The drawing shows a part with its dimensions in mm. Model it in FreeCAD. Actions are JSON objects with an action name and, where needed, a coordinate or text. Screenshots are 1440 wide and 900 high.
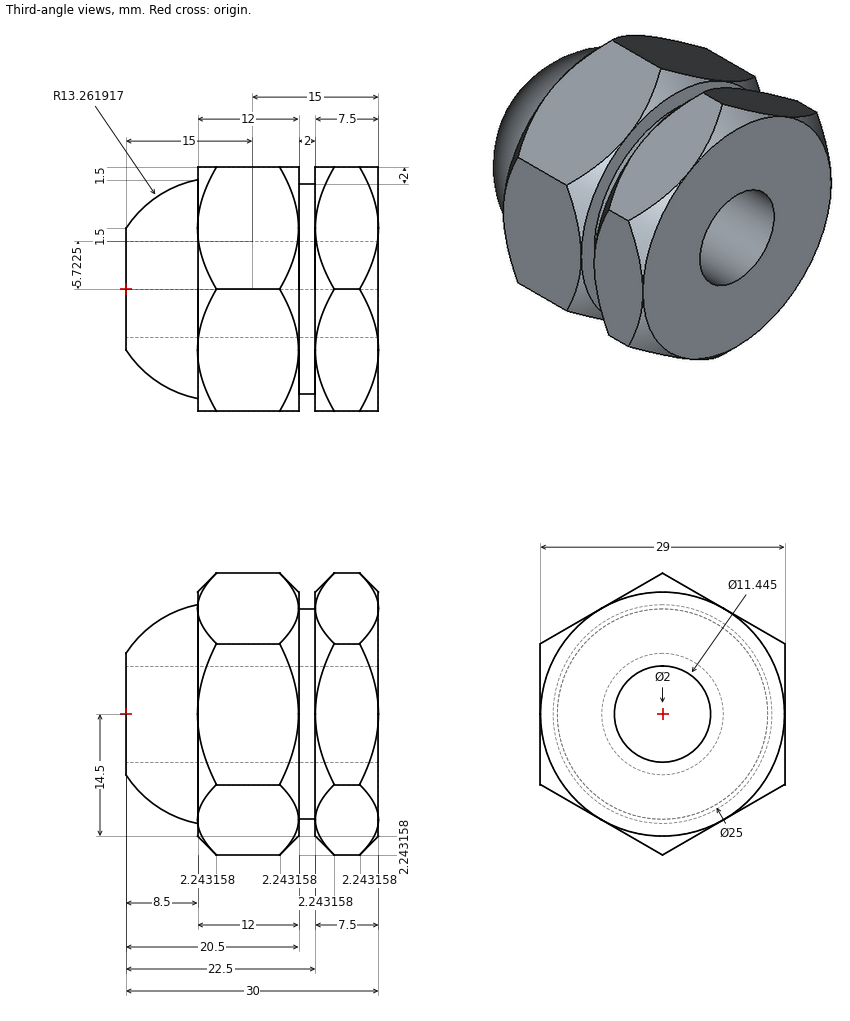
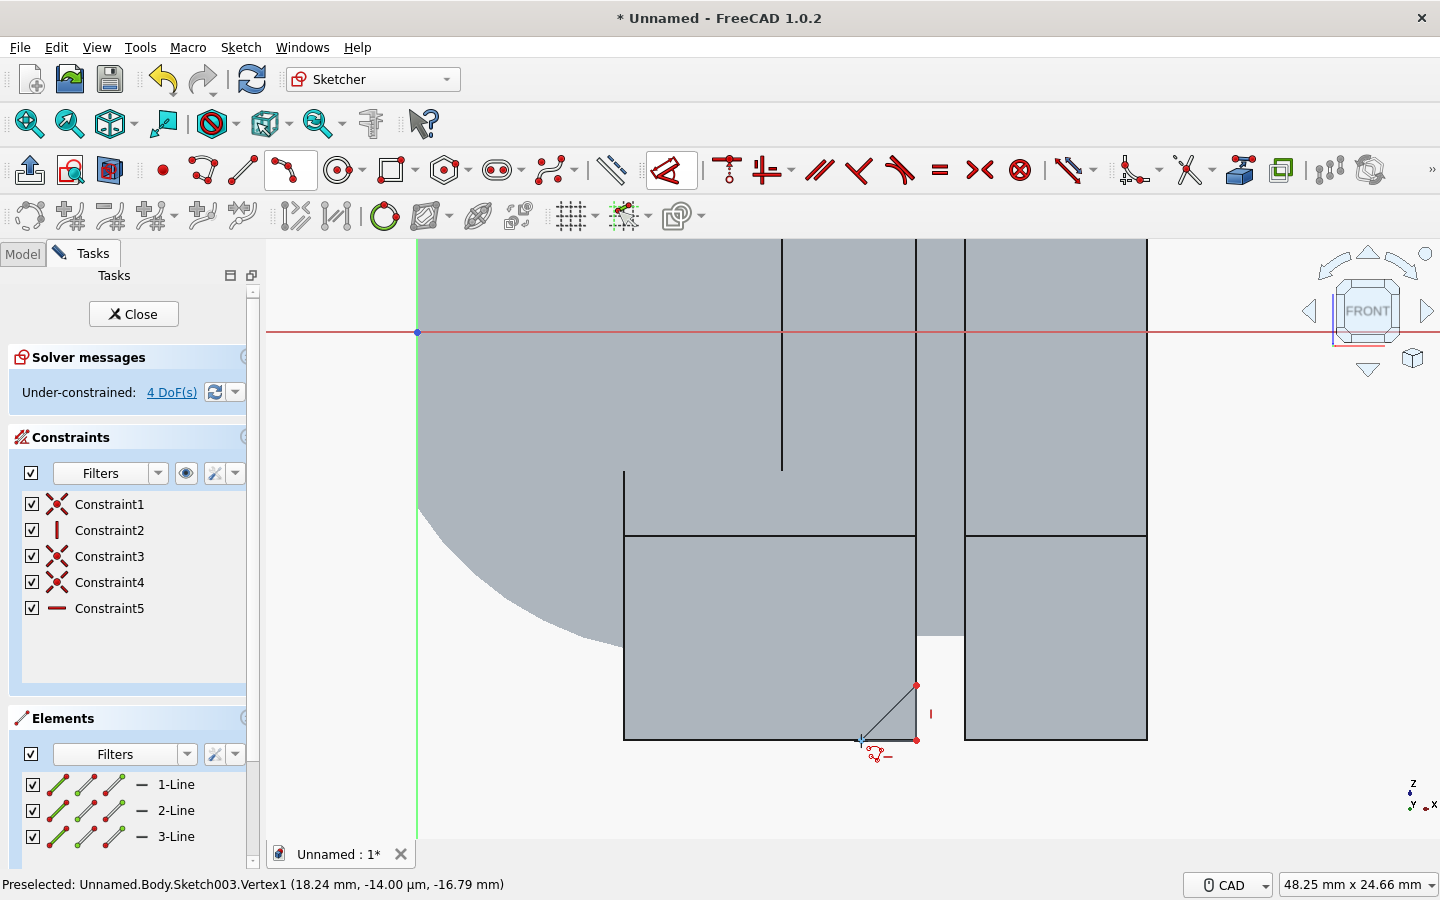
{"action": "left_click", "coordinate": [965, 685]}
{"action": "left_click", "coordinate": [1019, 740]}
{"action": "left_click", "coordinate": [965, 740]}
{"action": "left_click", "coordinate": [965, 686]}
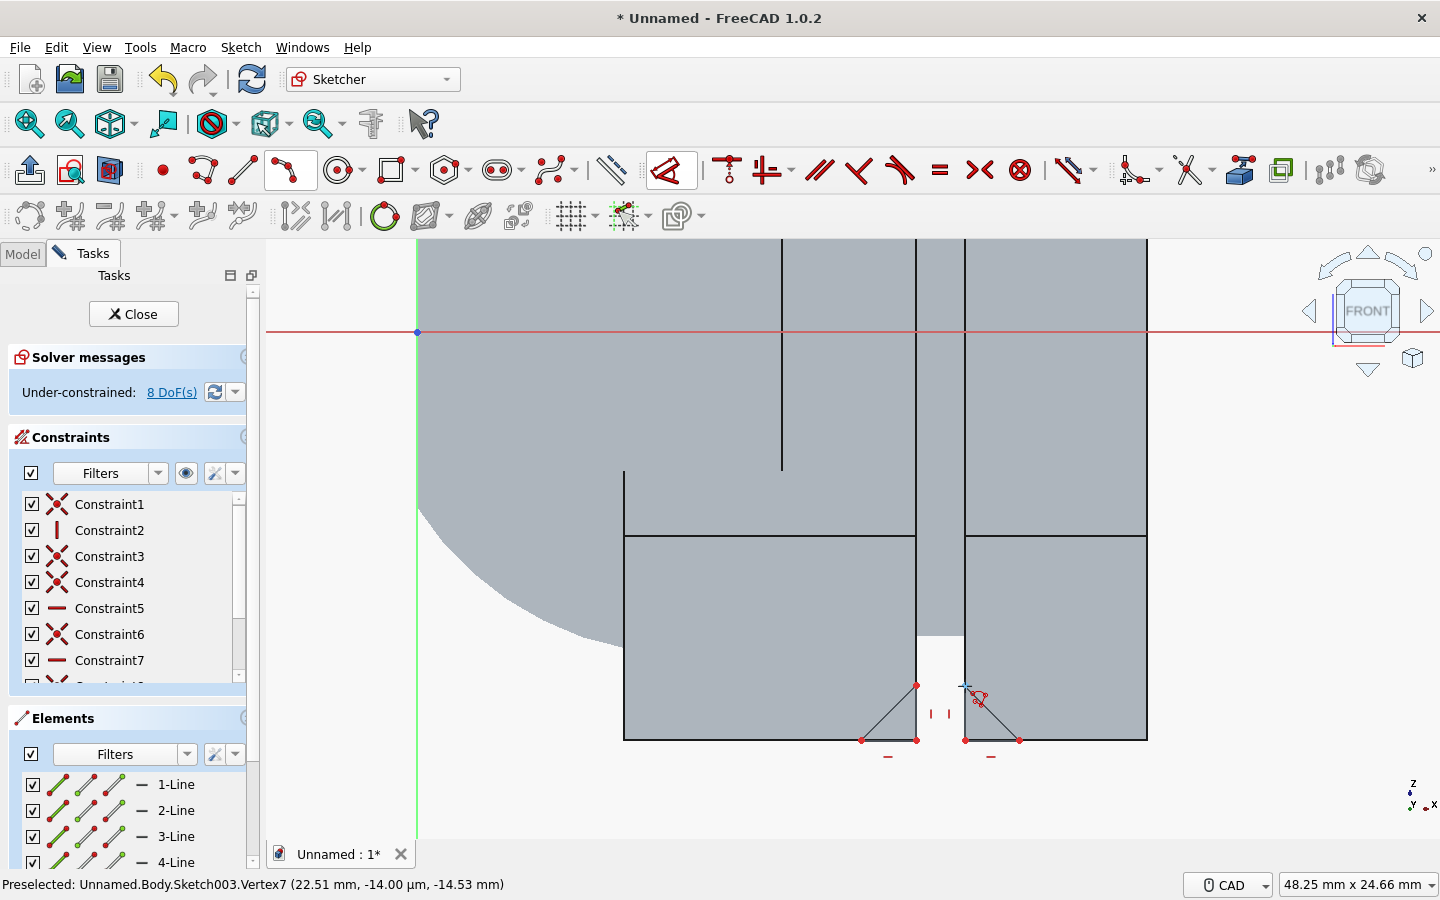
{"action": "left_click", "coordinate": [624, 685]}
{"action": "left_click", "coordinate": [679, 740]}
{"action": "left_click", "coordinate": [624, 740]}
{"action": "left_click", "coordinate": [624, 686]}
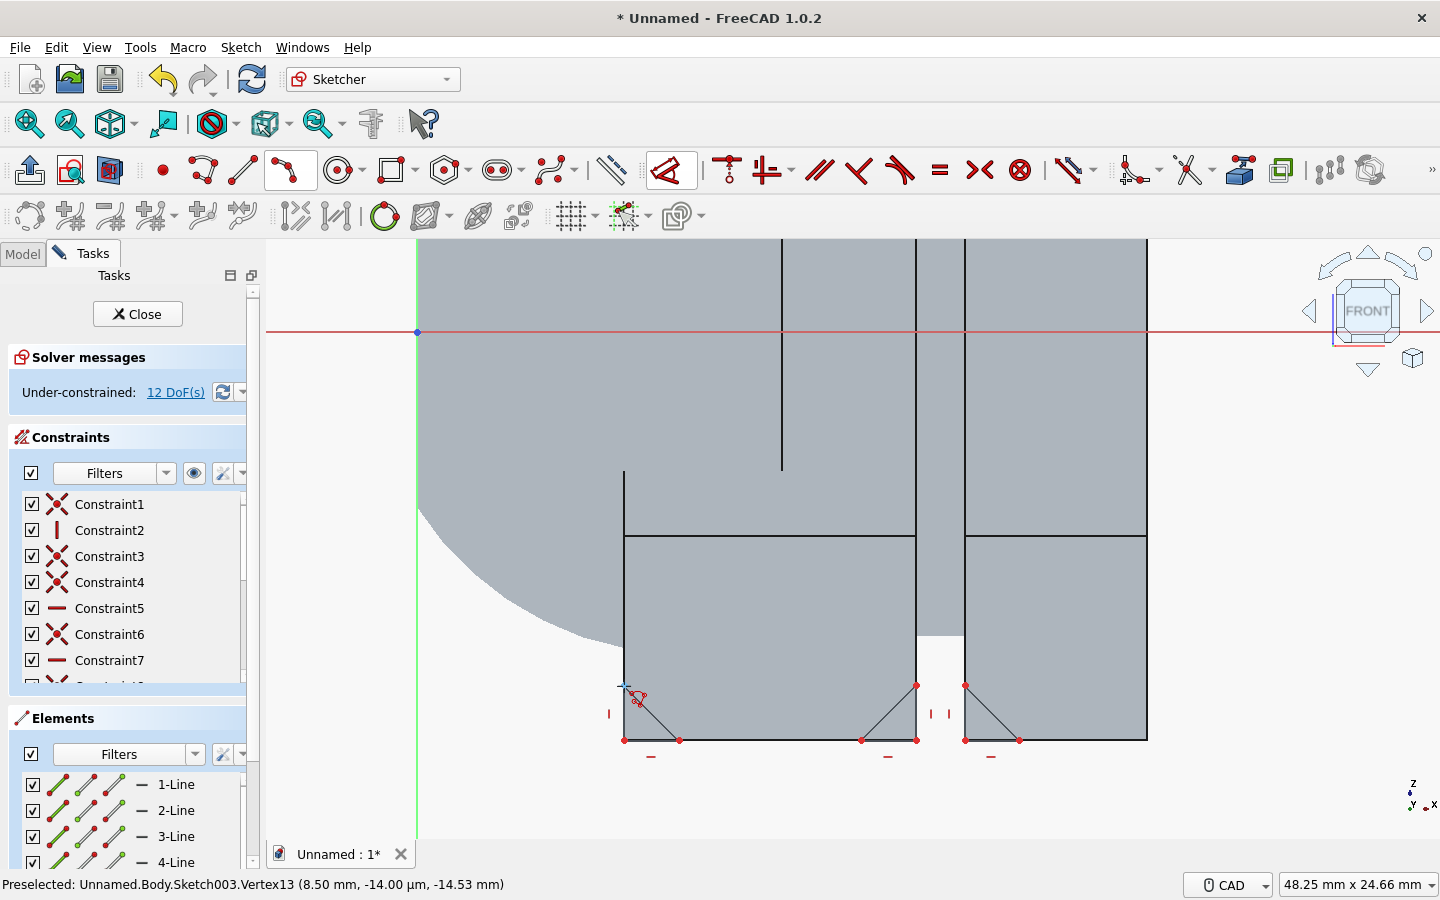
{"action": "left_click", "coordinate": [1093, 740]}
{"action": "left_click", "coordinate": [1147, 685]}
{"action": "left_click", "coordinate": [1147, 740]}
{"action": "left_click", "coordinate": [1093, 741]}
{"action": "key", "text": "Escape"}
{"action": "key", "text": "Escape"}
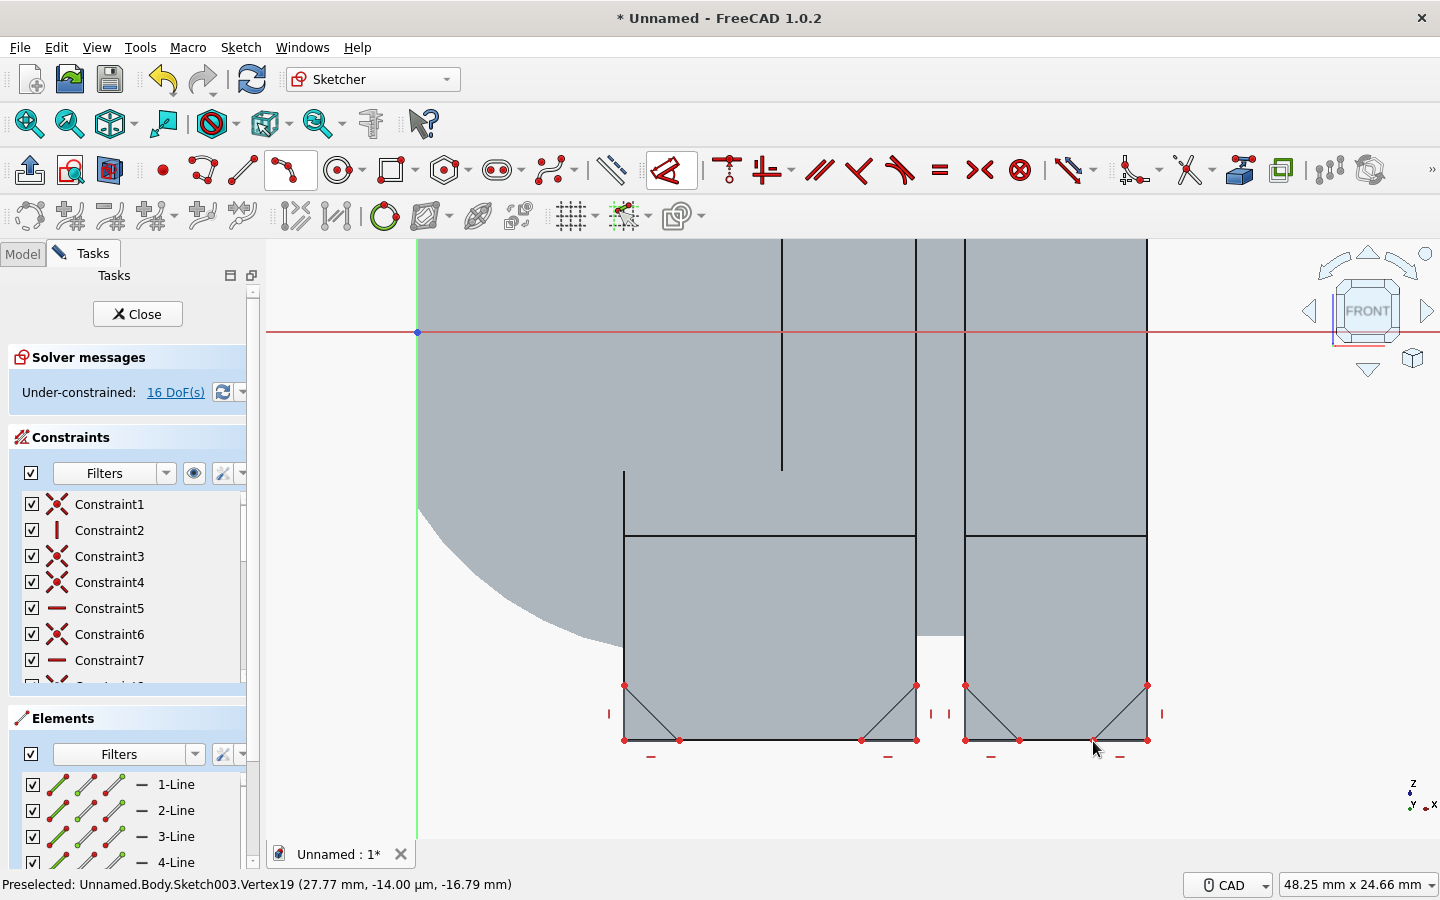
{"action": "left_click", "coordinate": [1147, 686]}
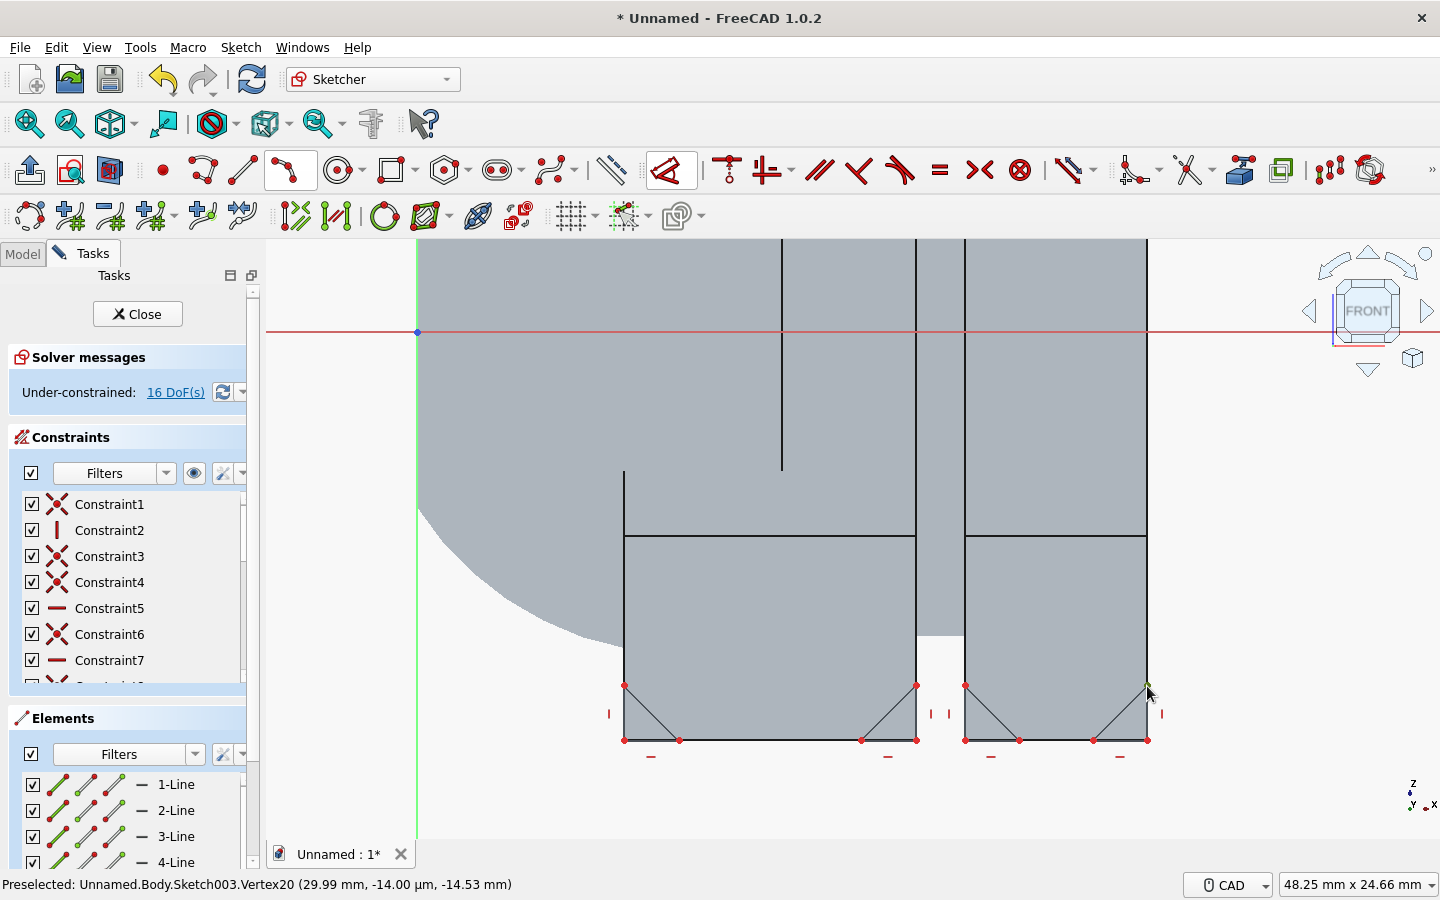
{"action": "key", "text": "l"}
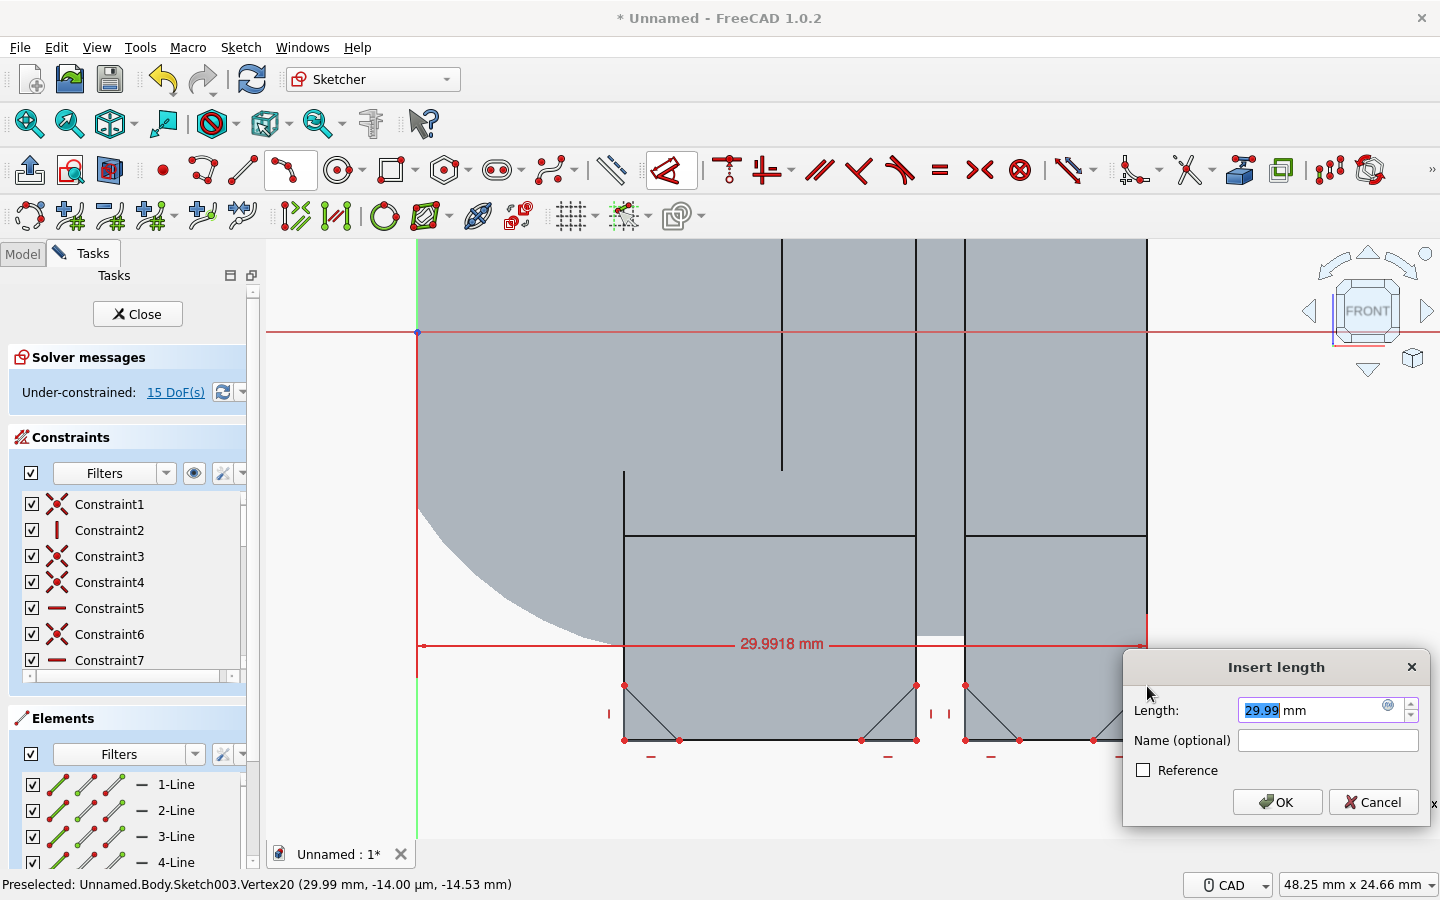
{"action": "type", "text": "30"}
{"action": "key", "text": "Return"}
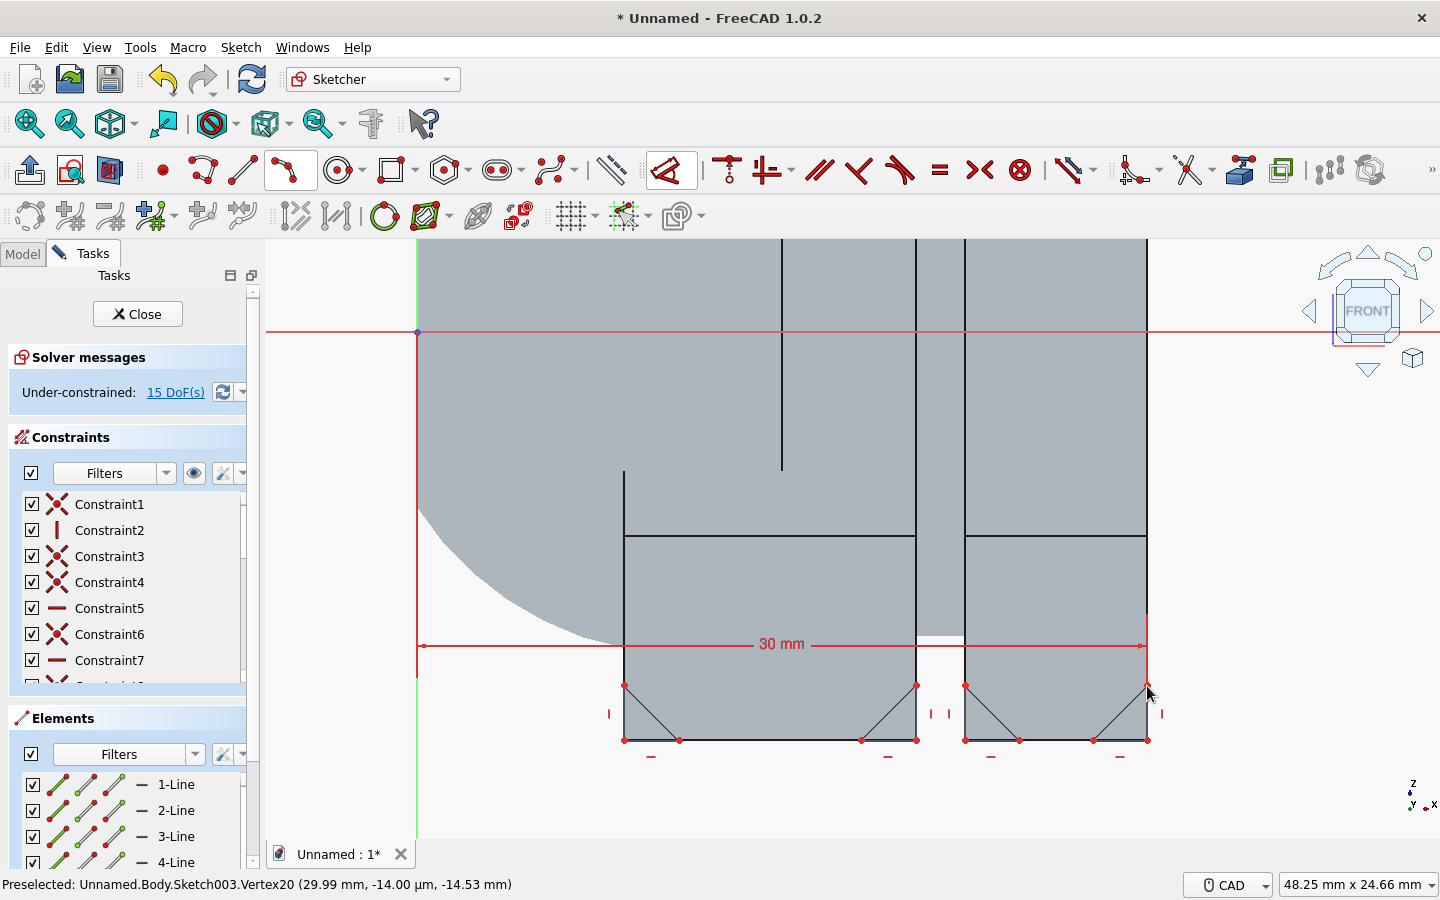
{"action": "left_click", "coordinate": [624, 686]}